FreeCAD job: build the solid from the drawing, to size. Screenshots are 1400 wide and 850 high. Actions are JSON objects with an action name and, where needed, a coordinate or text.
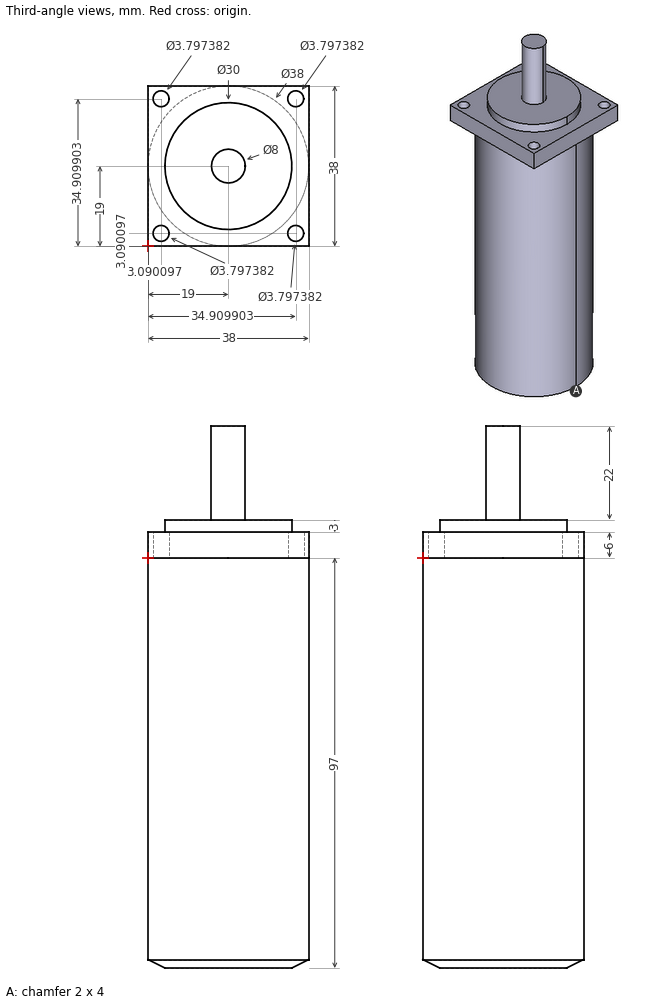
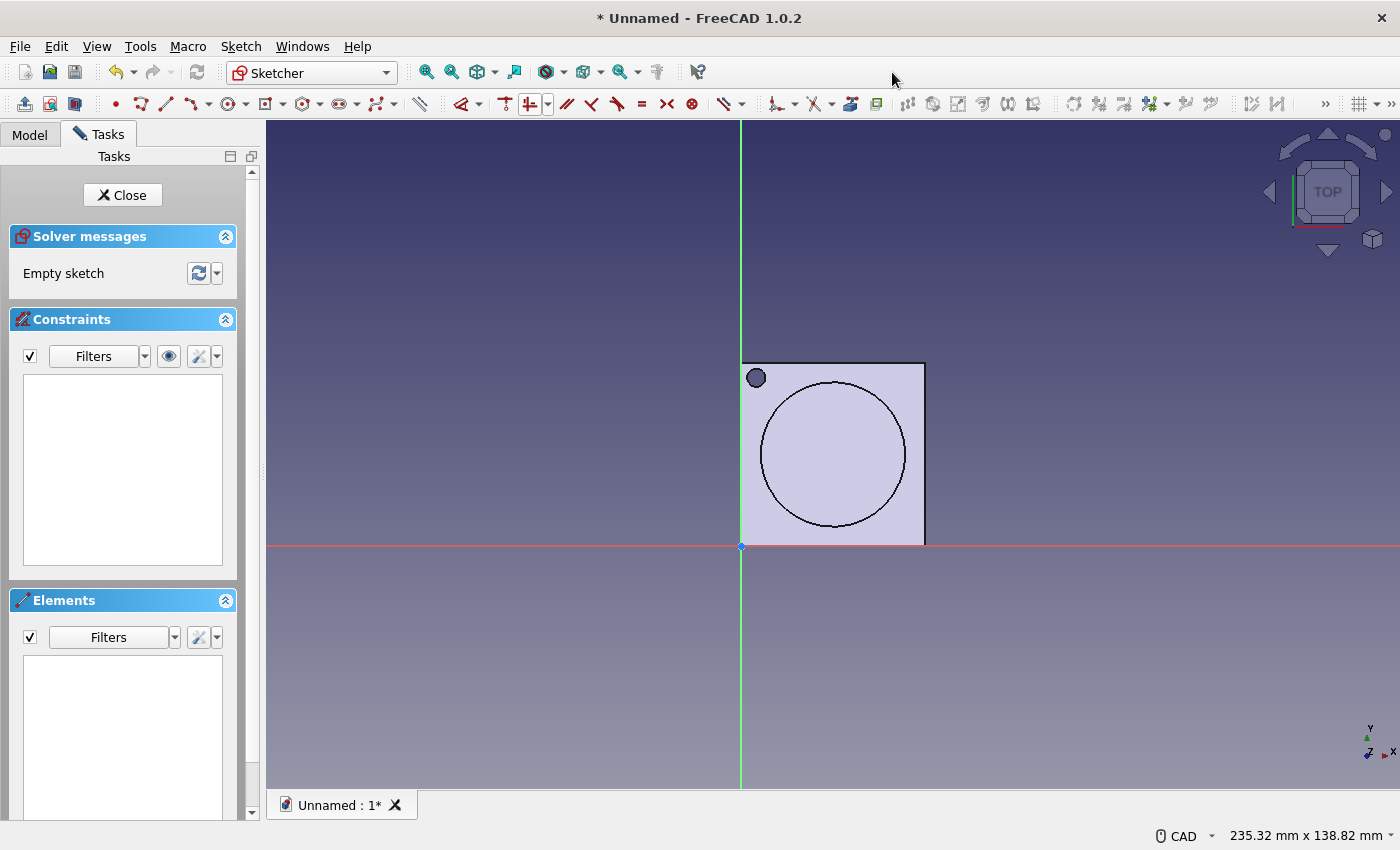
{"action": "scroll", "coordinate": [917, 374], "scroll_direction": "up", "scroll_amount": 15}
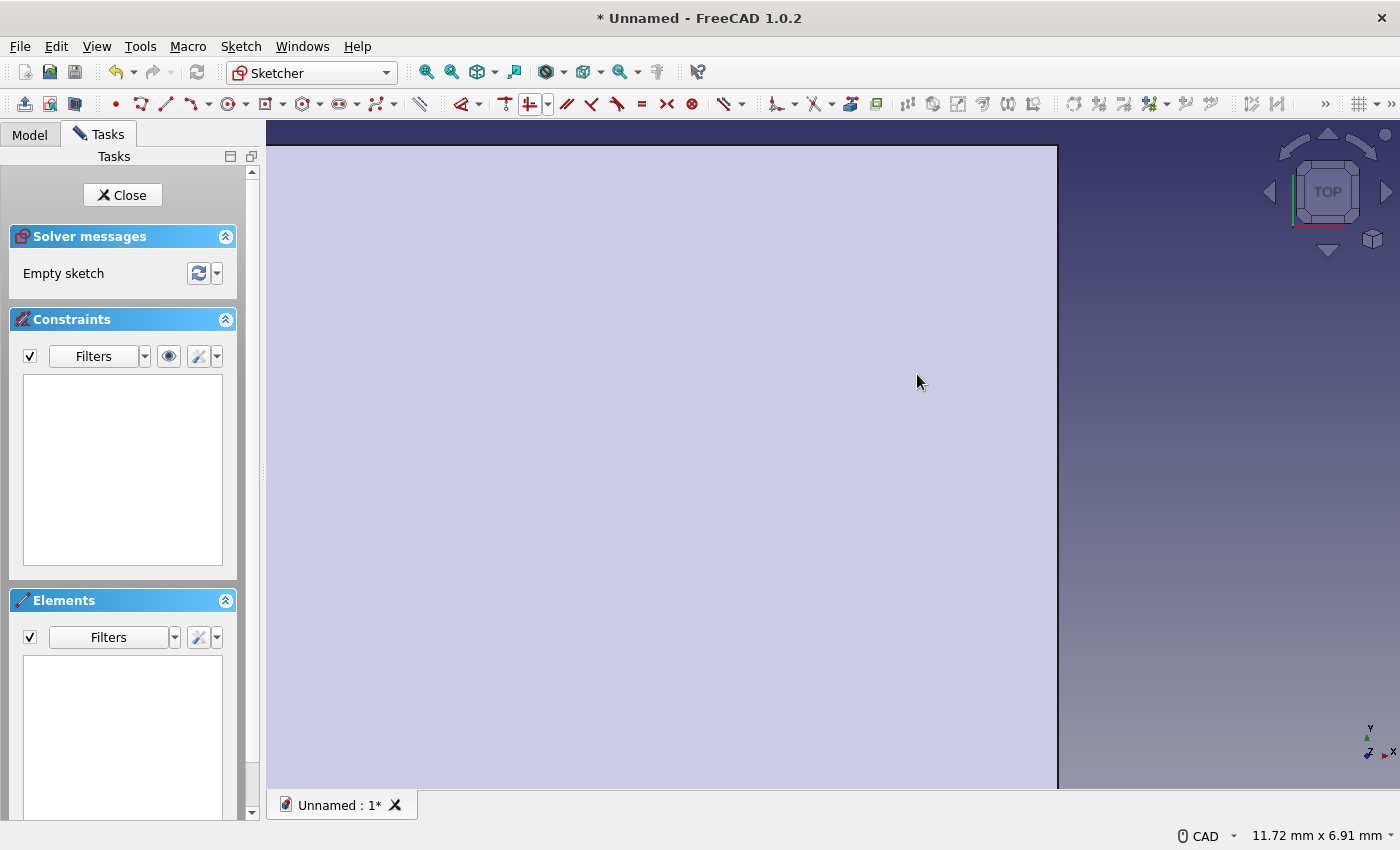
{"action": "left_click", "coordinate": [228, 104]}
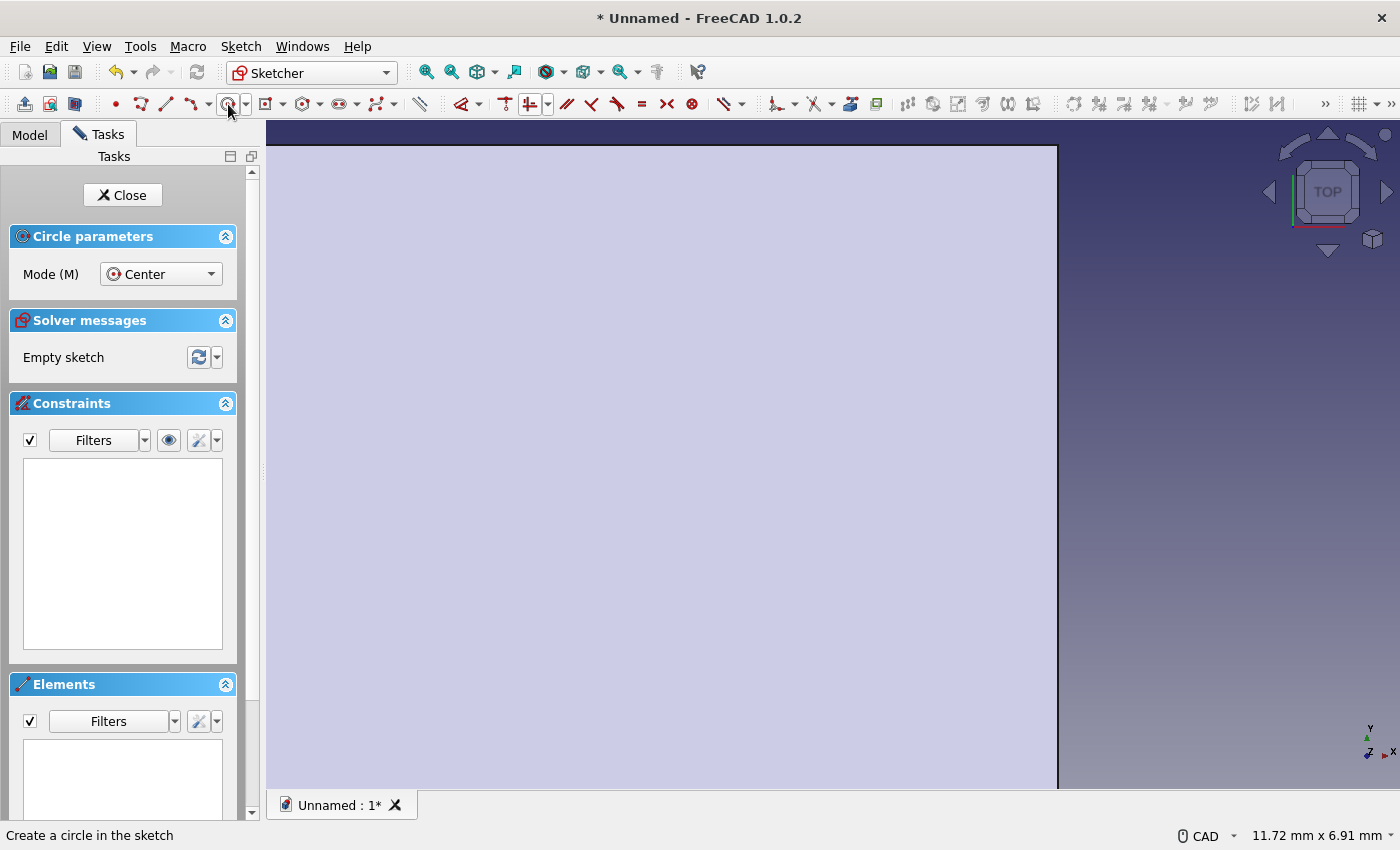
{"action": "left_click", "coordinate": [759, 444]}
{"action": "mouse_move", "coordinate": [889, 314]}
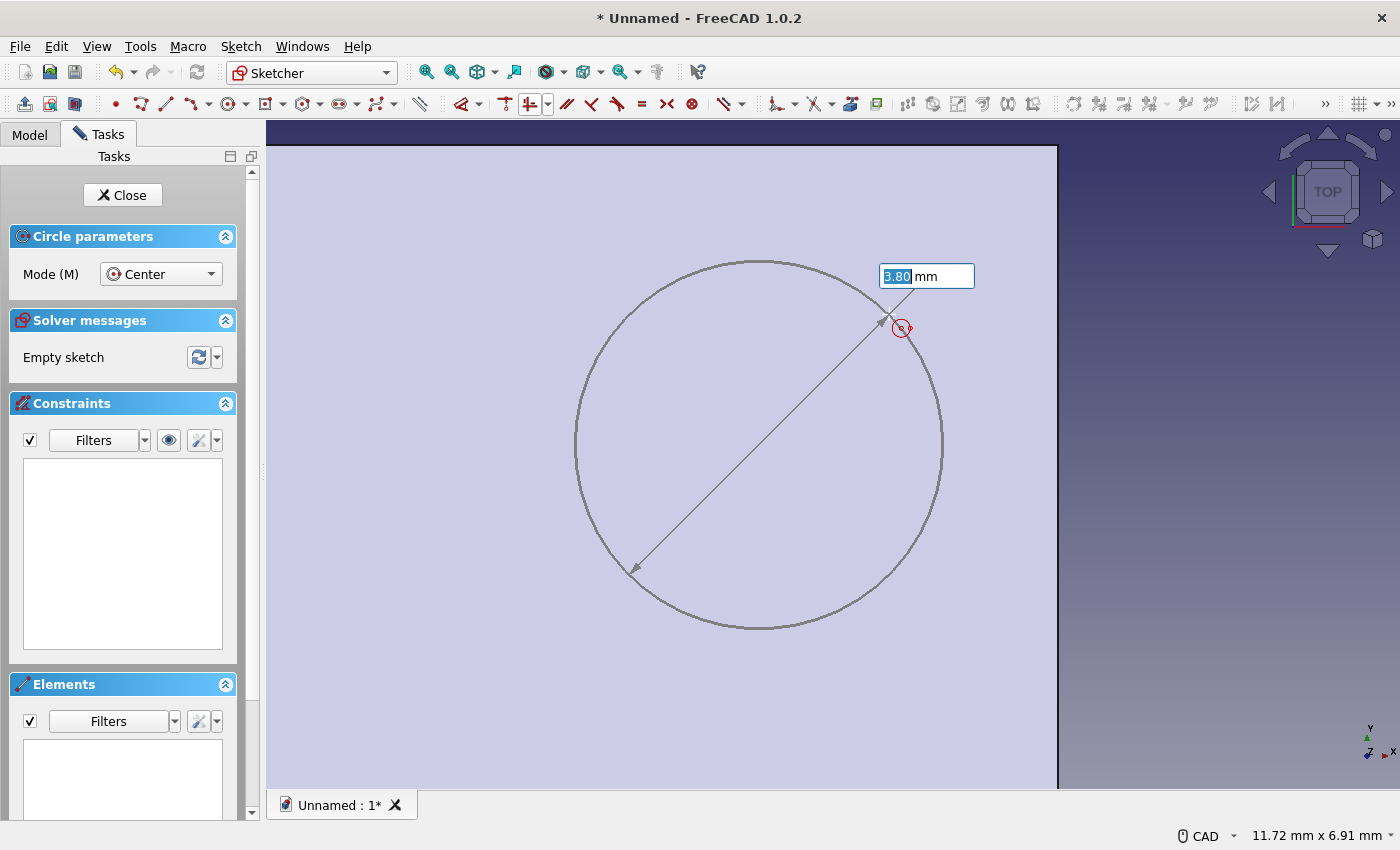
{"action": "type", "text": "3.797382"}
{"action": "key", "text": "Return"}
{"action": "key", "text": "Escape"}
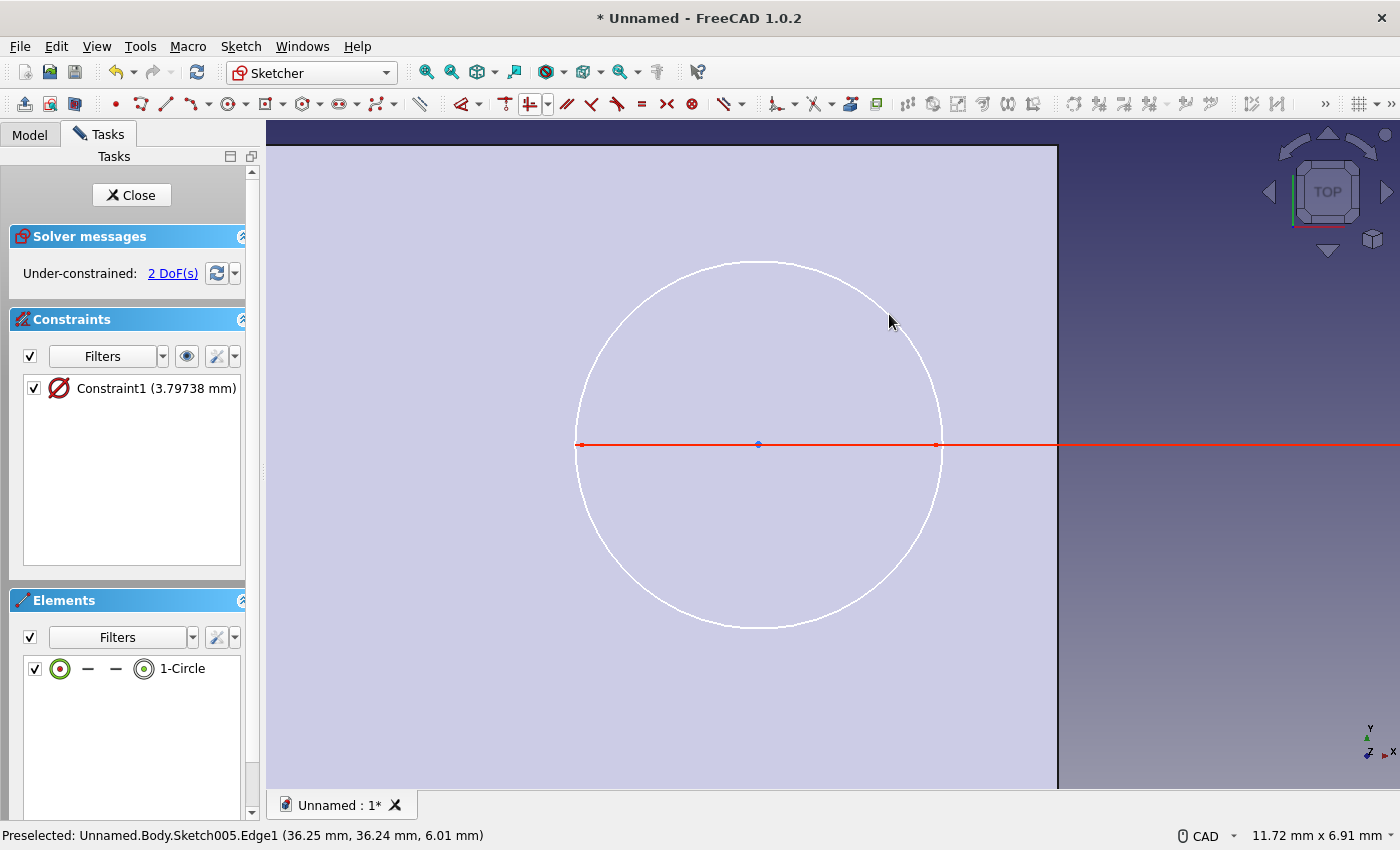
{"action": "left_click", "coordinate": [460, 104]}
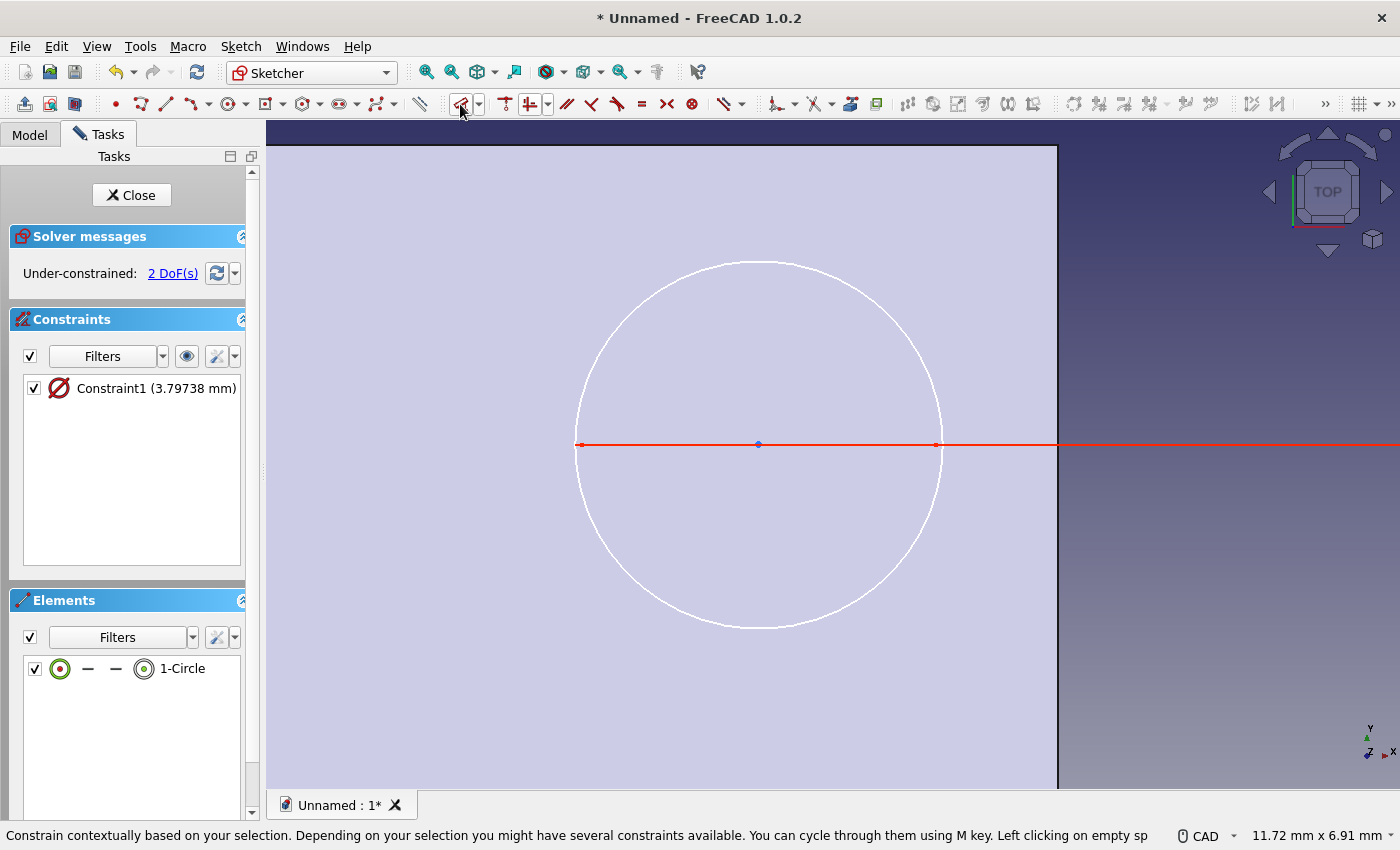
{"action": "left_click", "coordinate": [759, 445]}
{"action": "left_click", "coordinate": [526, 411]}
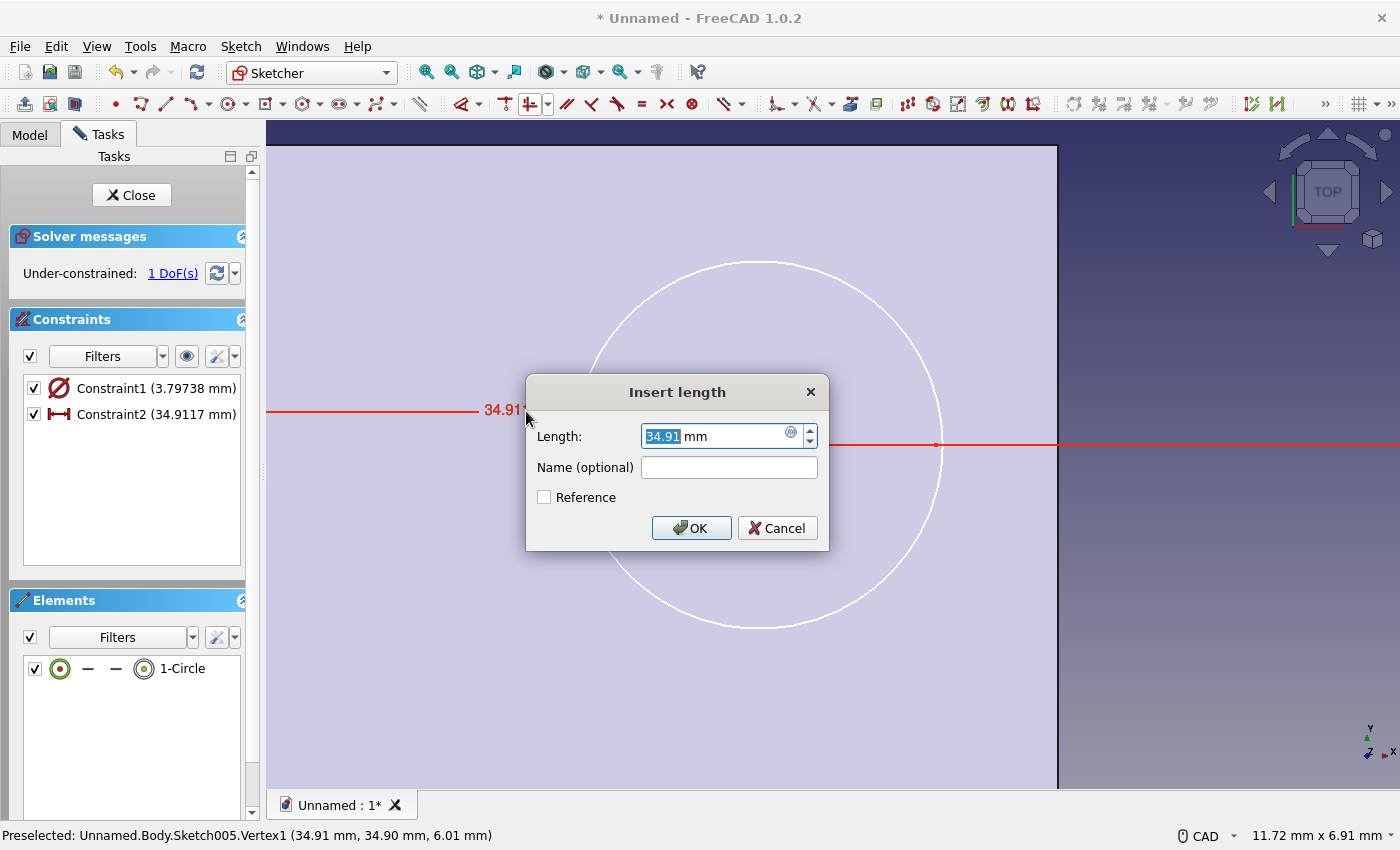
{"action": "type", "text": "34.909903"}
{"action": "key", "text": "Return"}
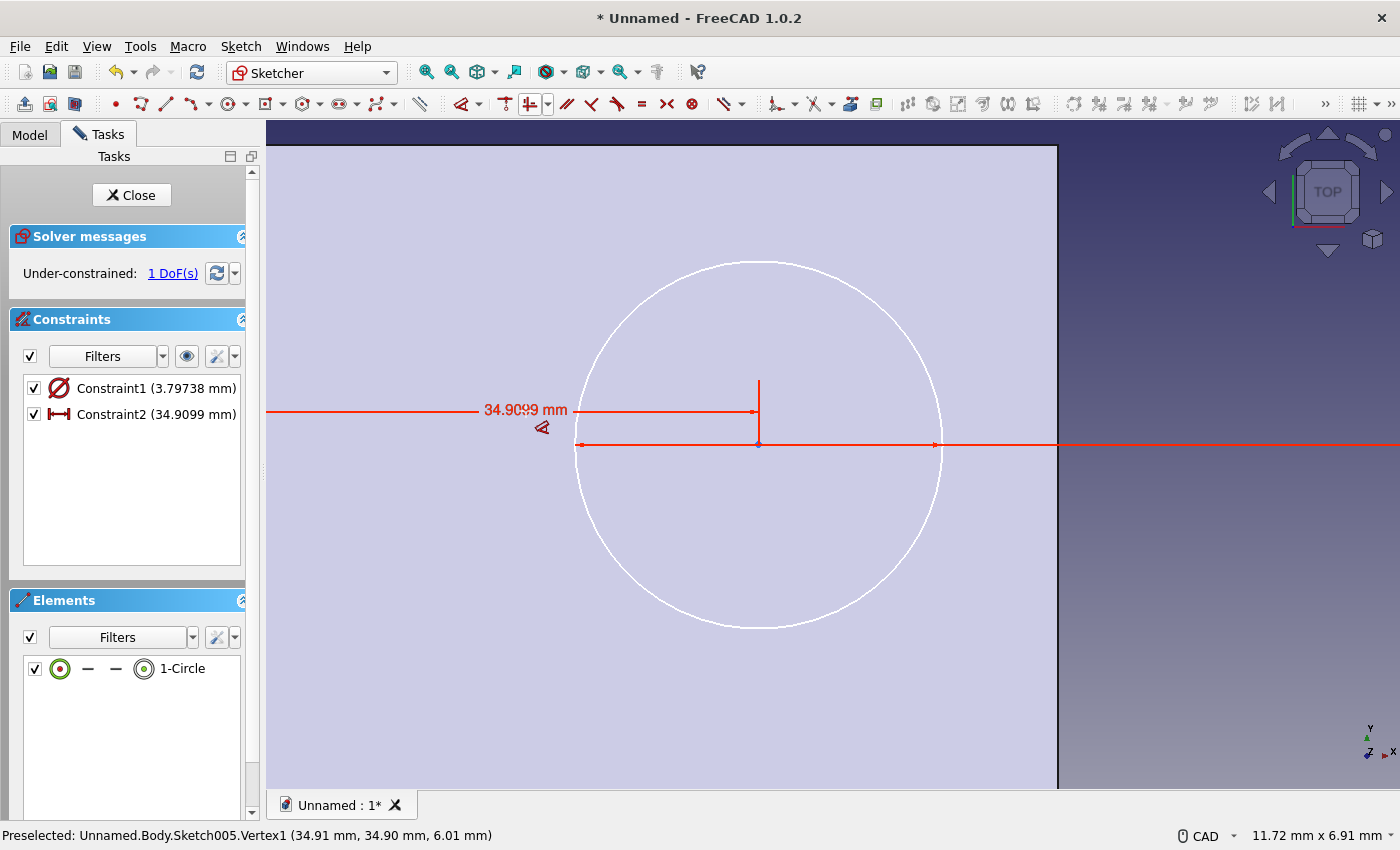
{"action": "left_click", "coordinate": [759, 445]}
{"action": "left_click", "coordinate": [793, 603]}